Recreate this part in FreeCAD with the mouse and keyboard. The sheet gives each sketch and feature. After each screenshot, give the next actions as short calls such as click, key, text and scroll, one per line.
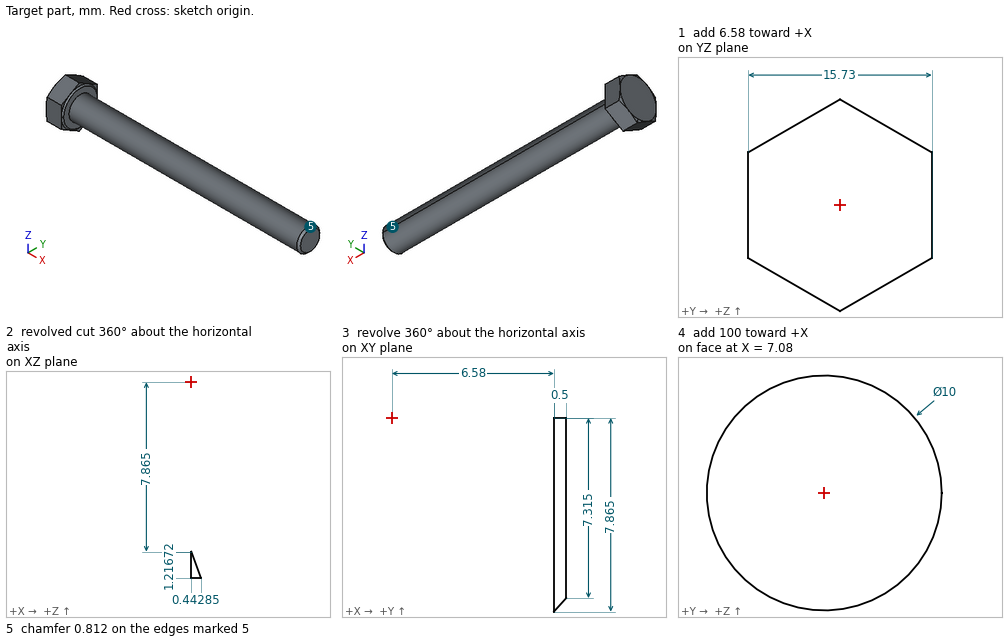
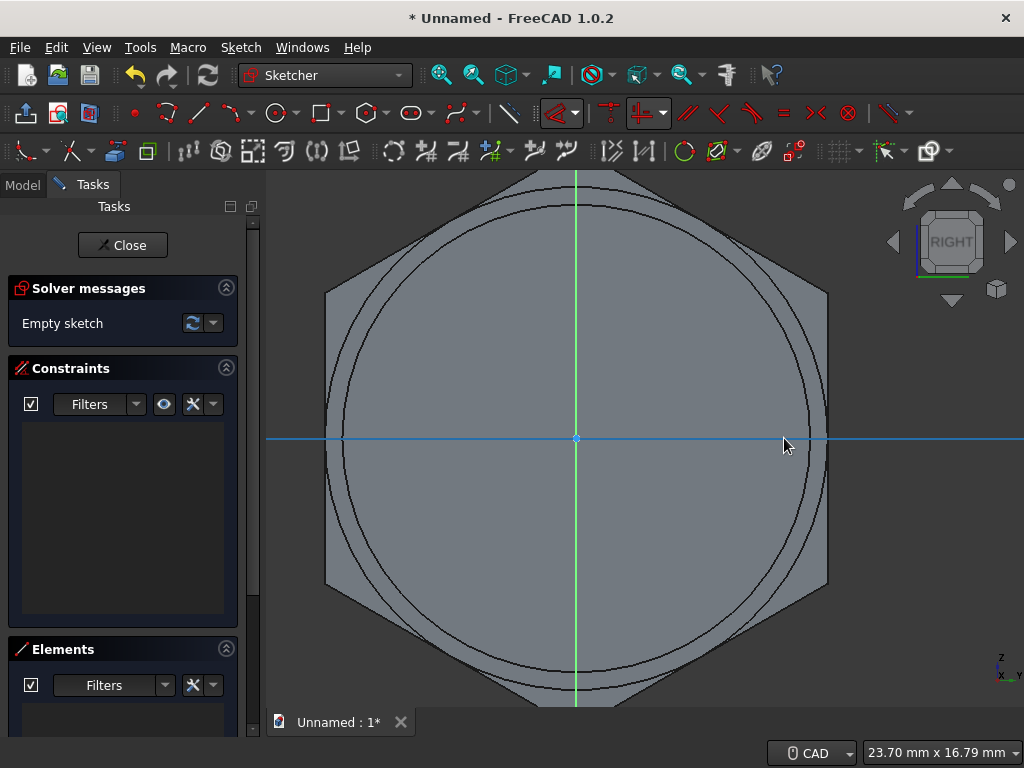
click(276, 114)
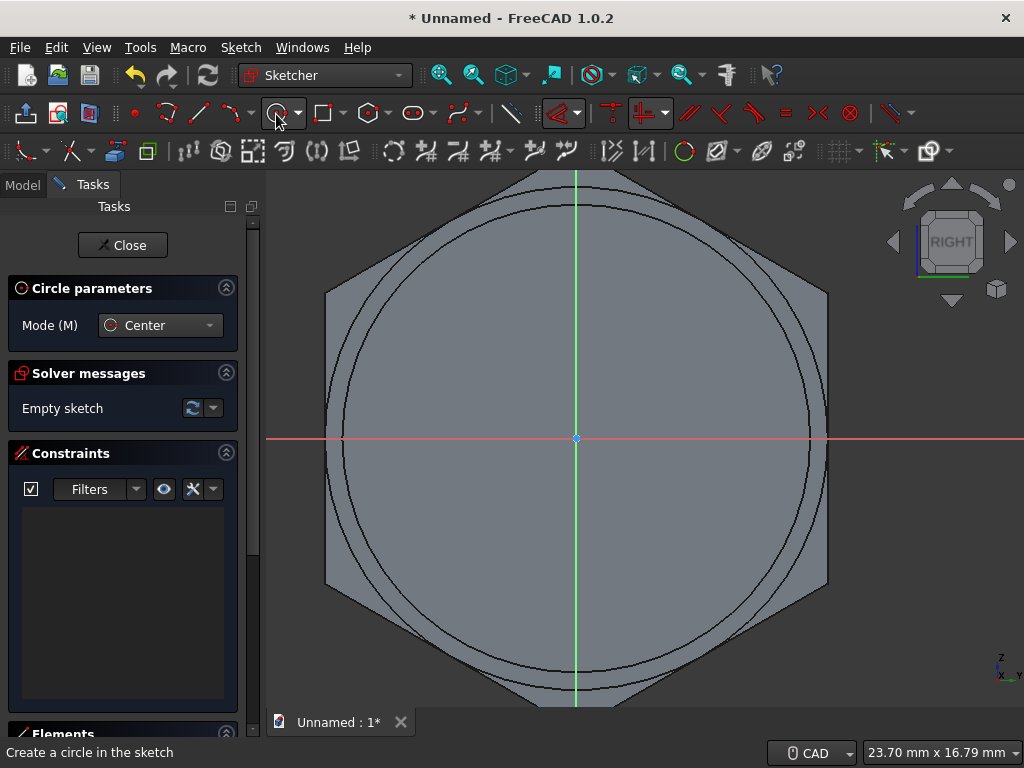
click(576, 438)
click(689, 325)
key(Escape)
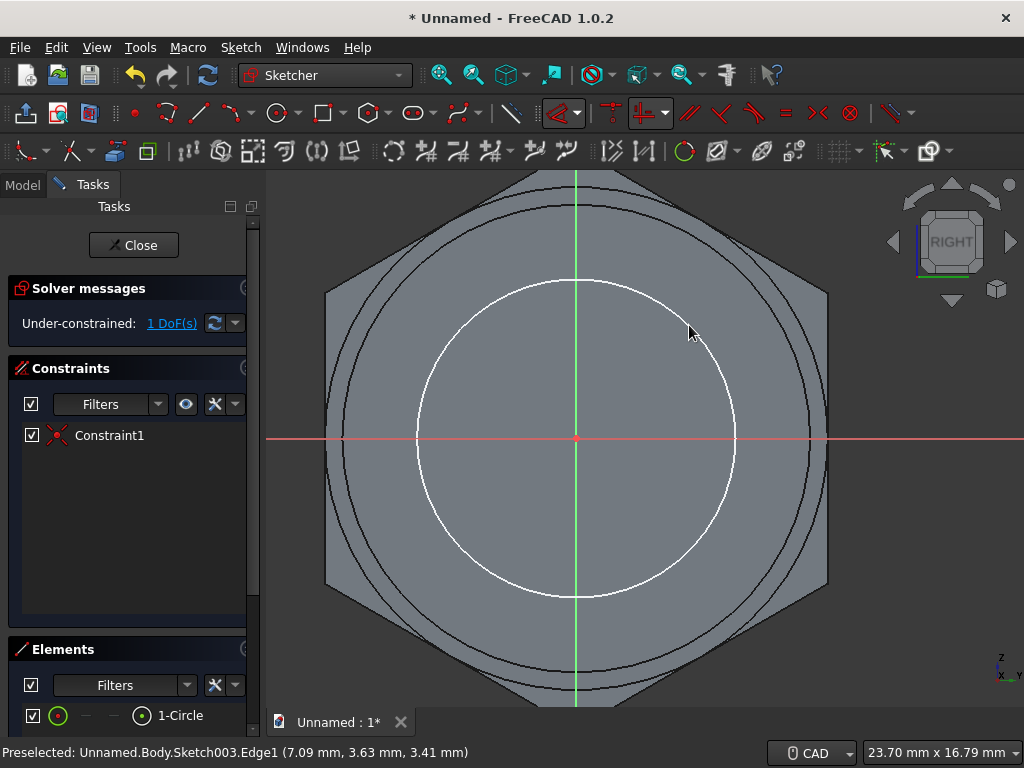
key(d)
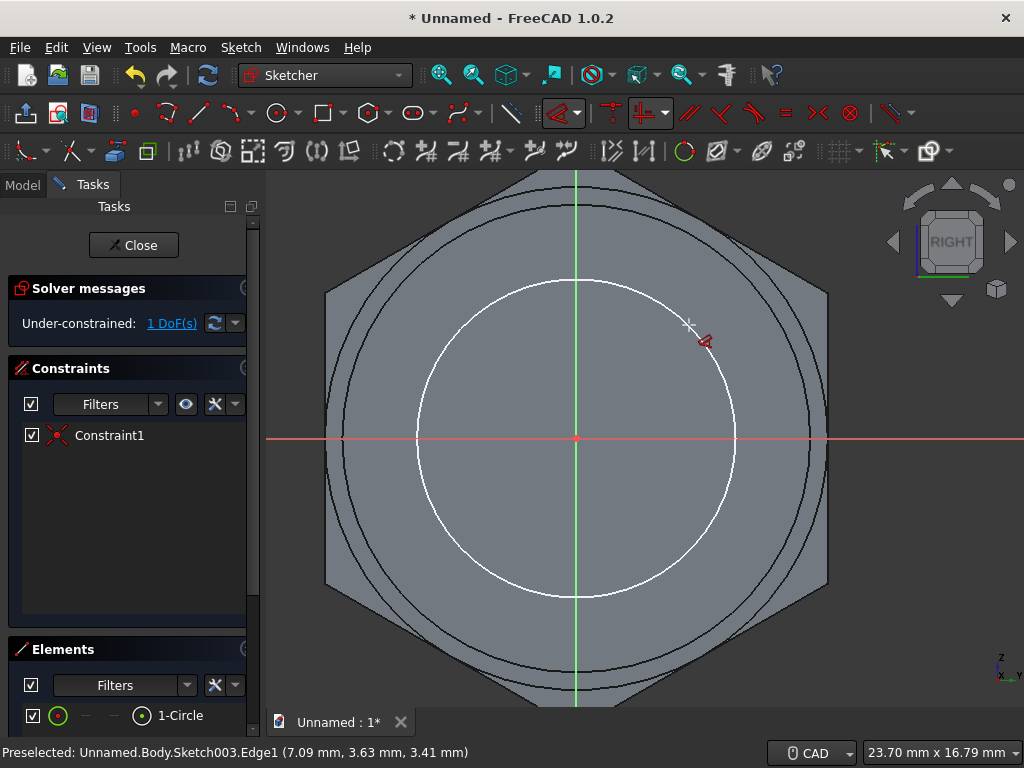
click(689, 326)
click(712, 303)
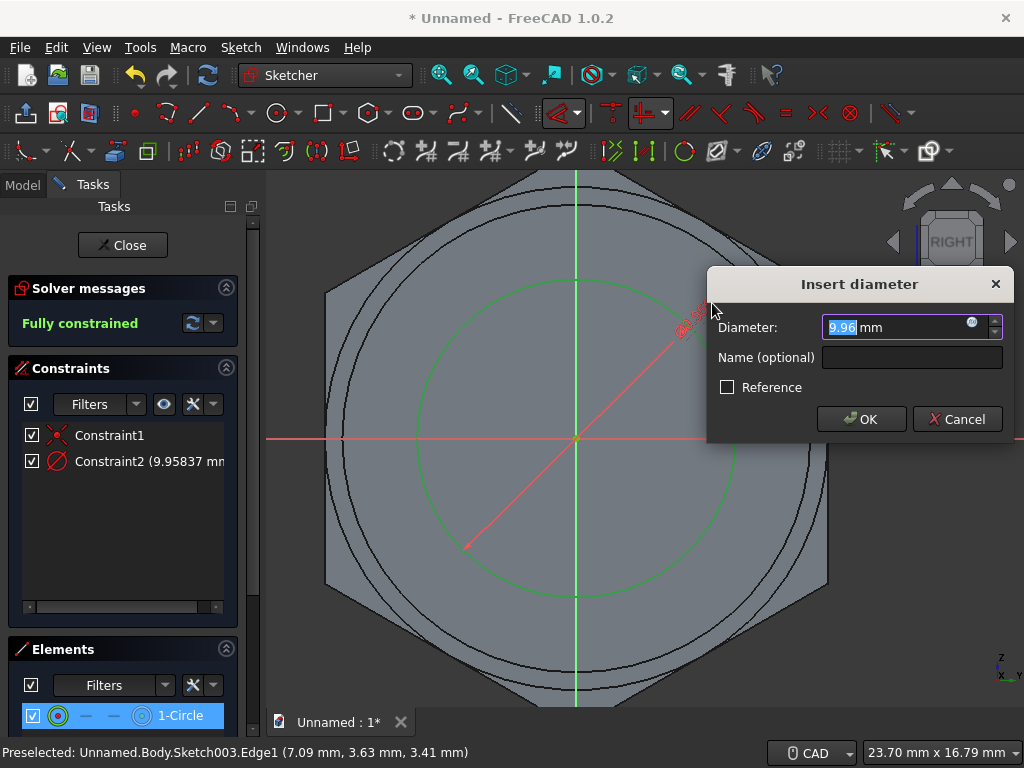
text(10)
key(Return)
key(Escape)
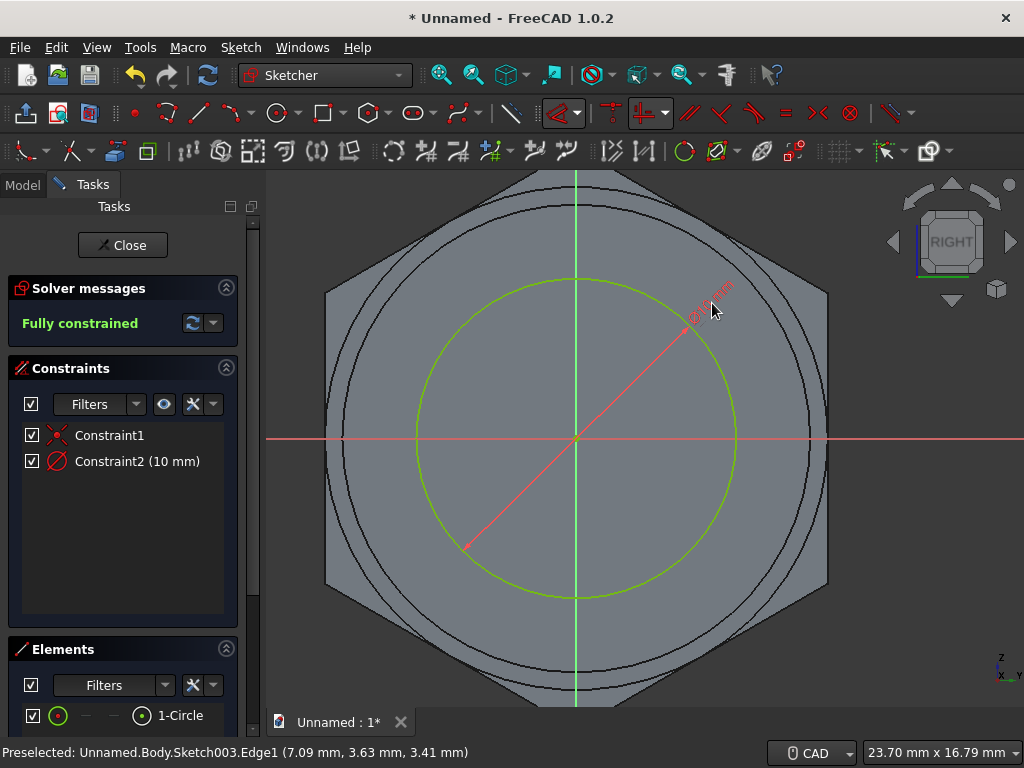
click(123, 245)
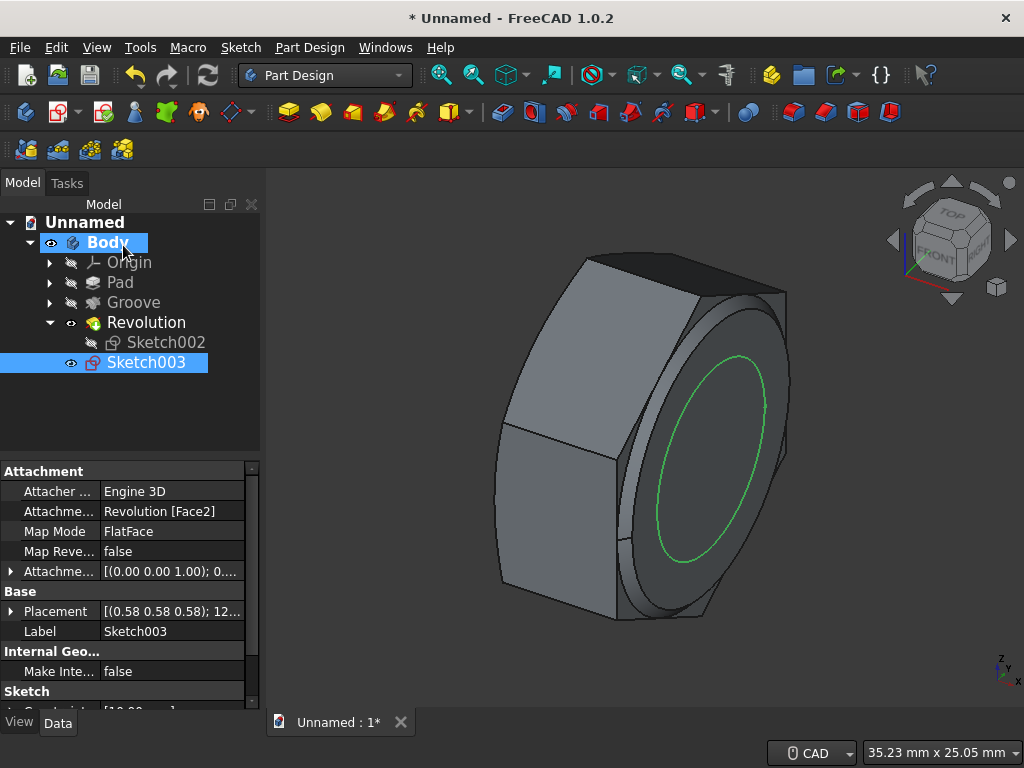
click(290, 112)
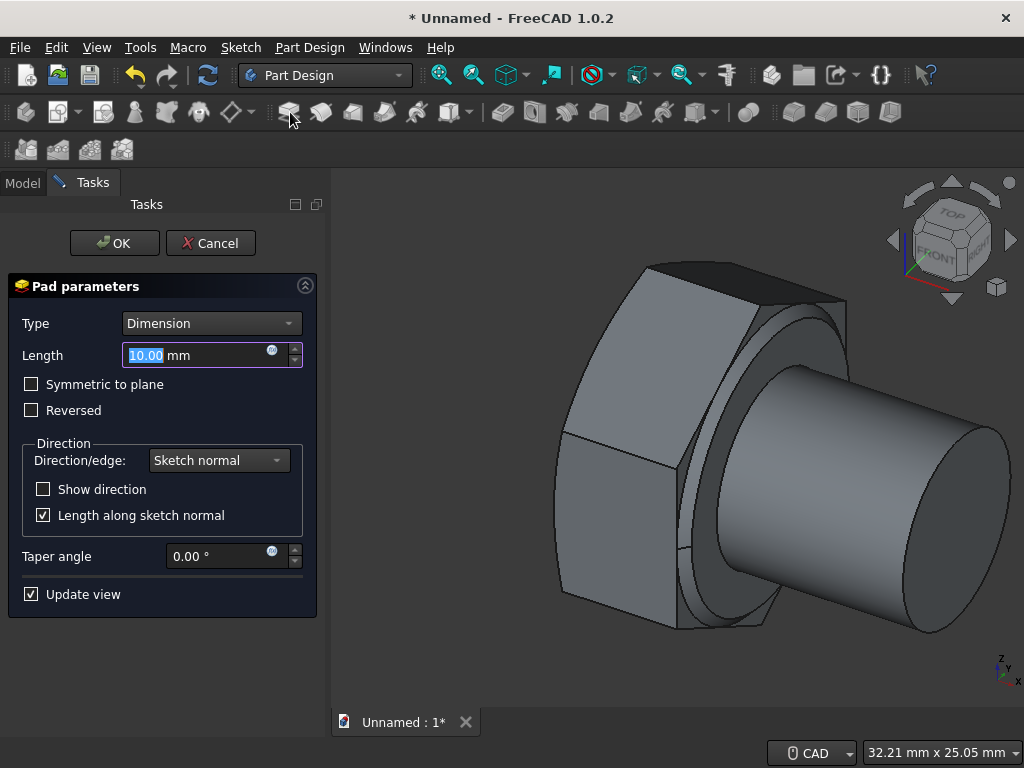
text(100)
key(Tab)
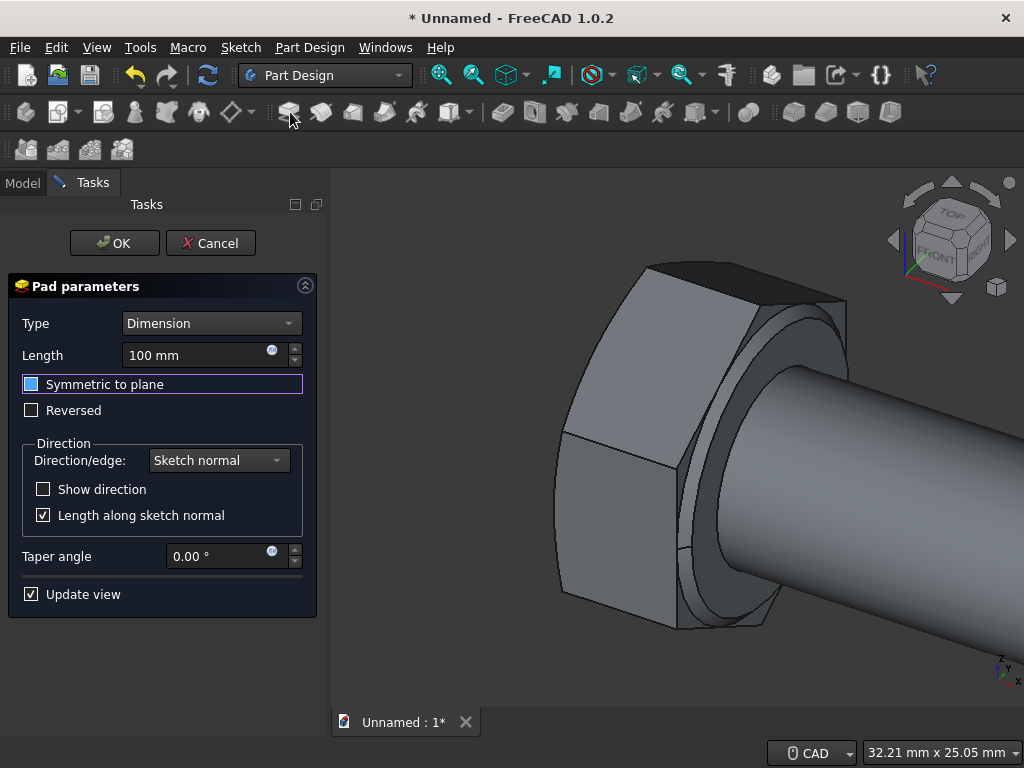
click(115, 243)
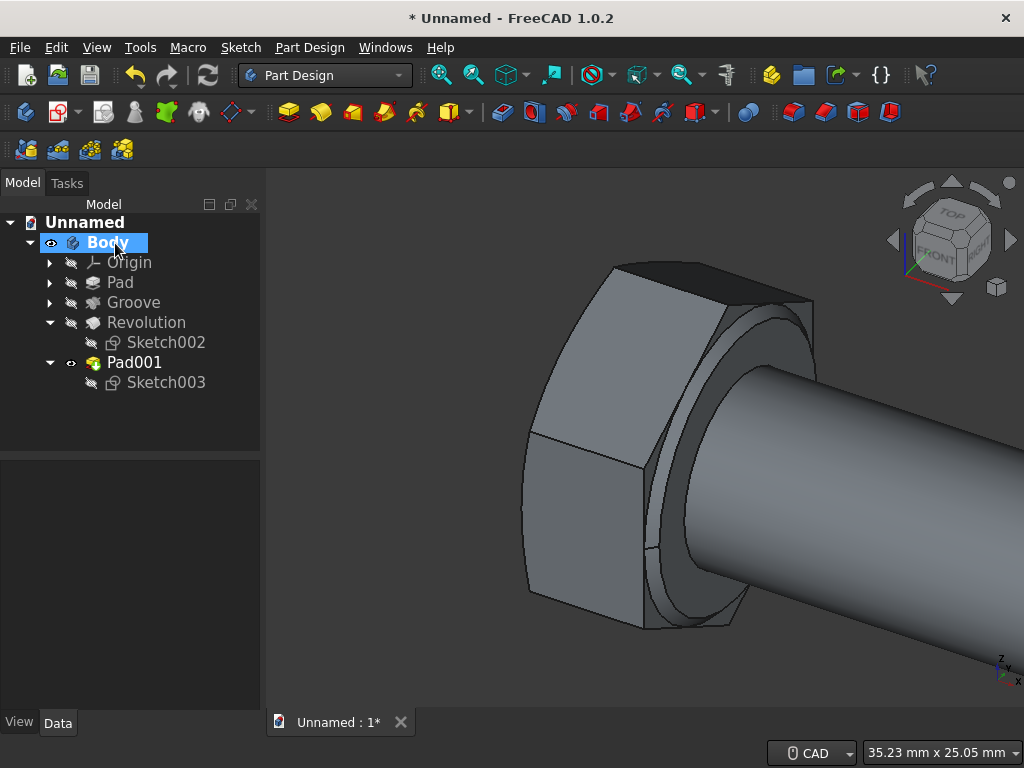
click(442, 76)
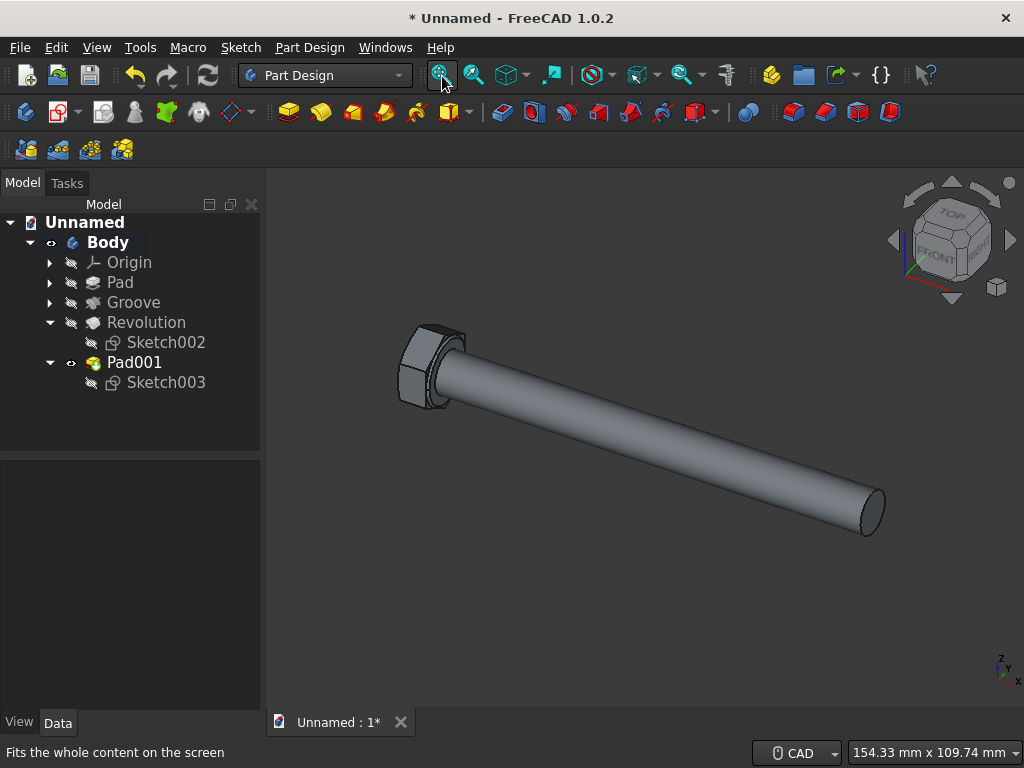
click(860, 524)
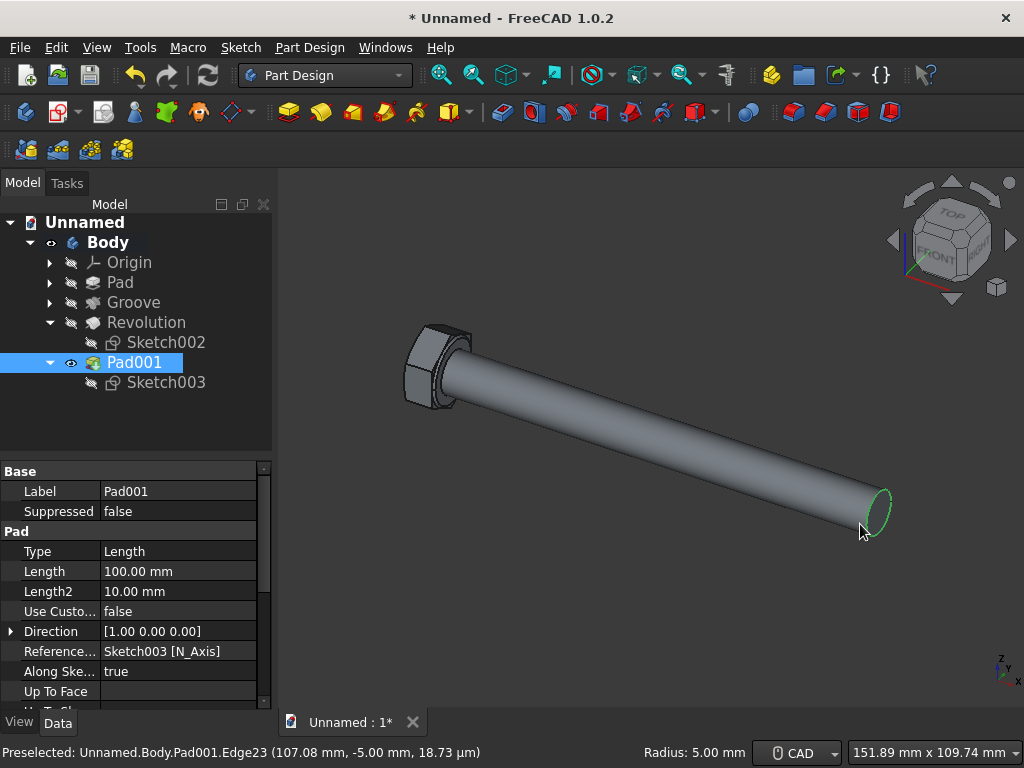
click(826, 112)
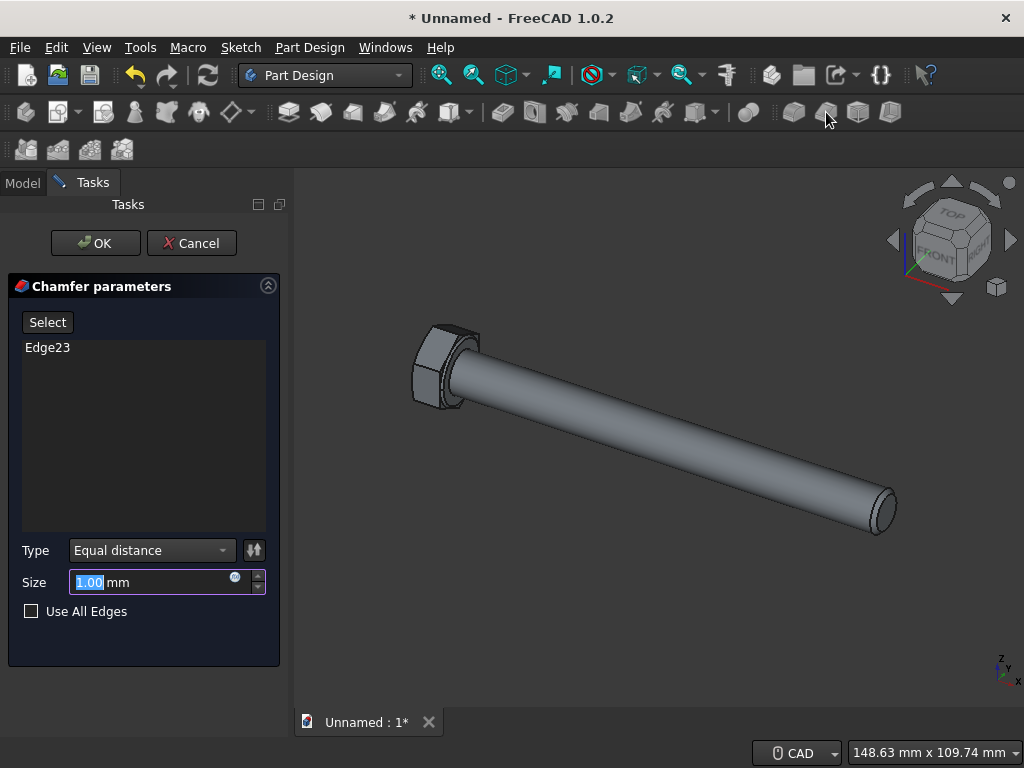
text(0.812)
key(Tab)